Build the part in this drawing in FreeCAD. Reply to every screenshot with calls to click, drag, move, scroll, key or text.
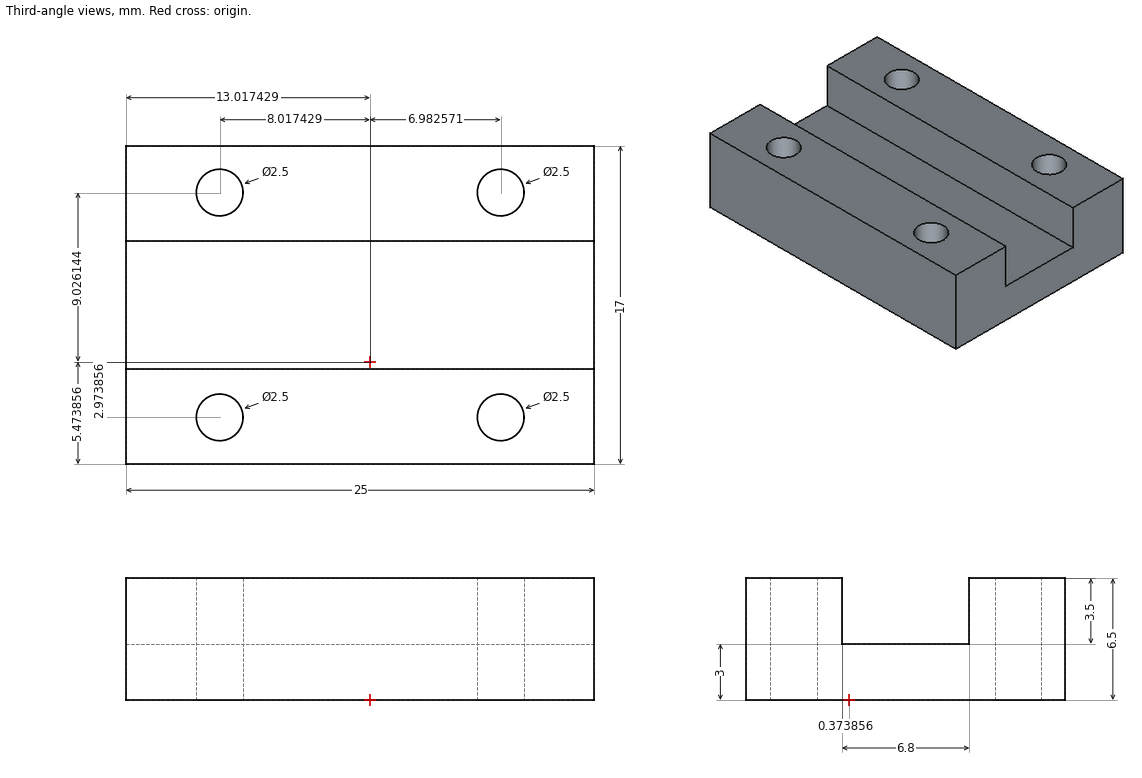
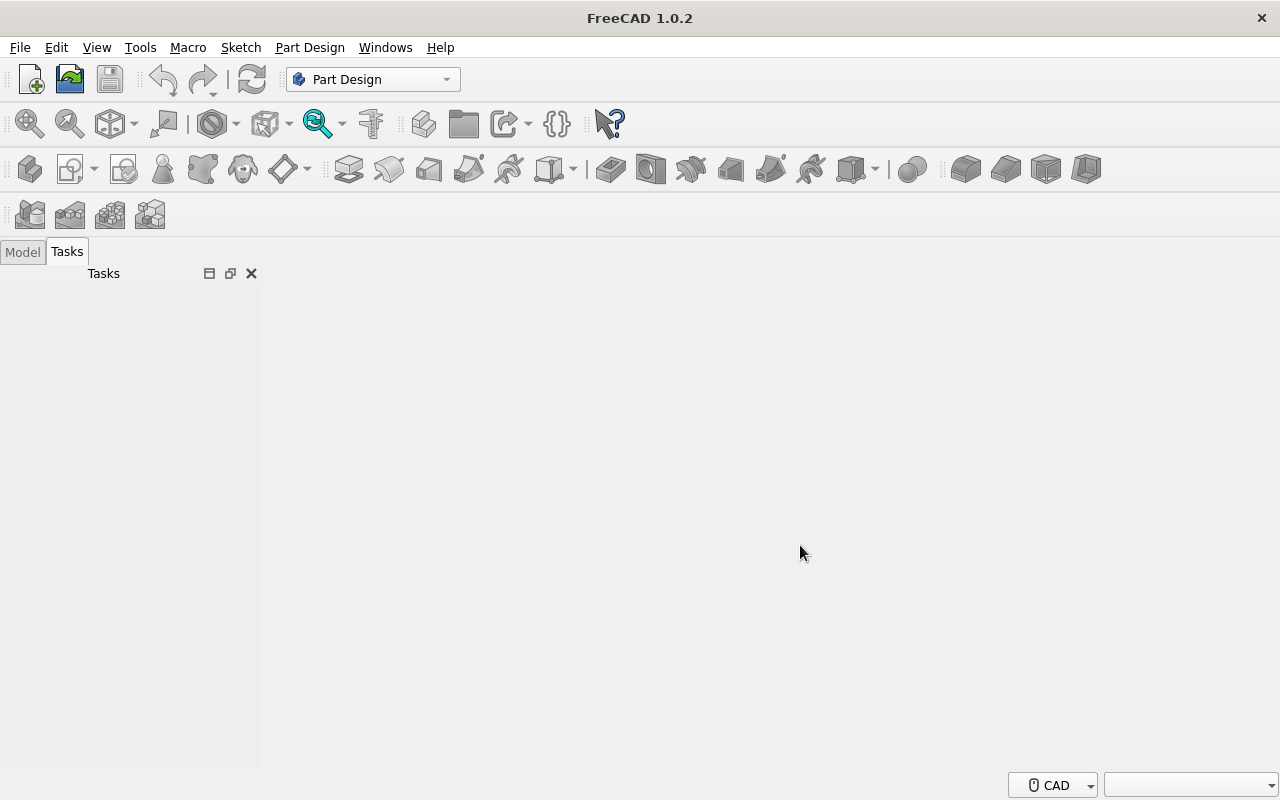
click(30, 80)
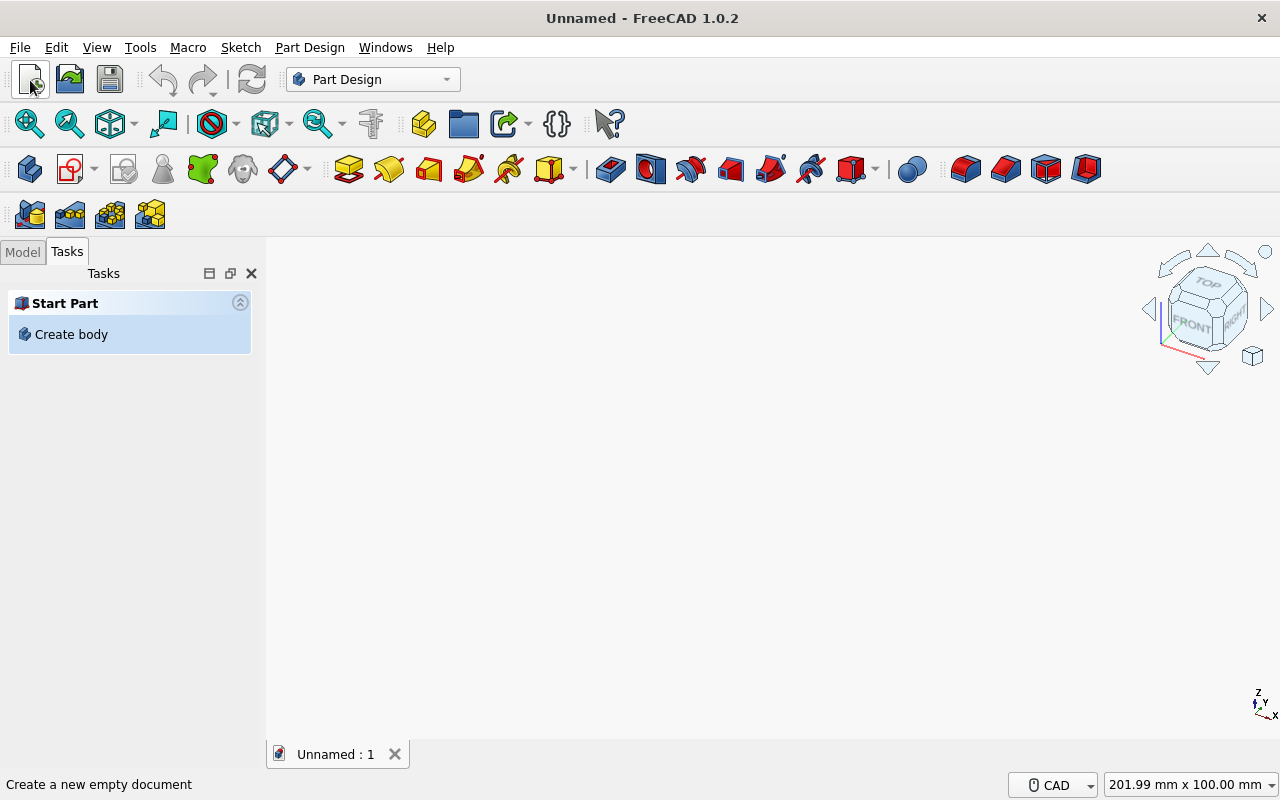
click(70, 170)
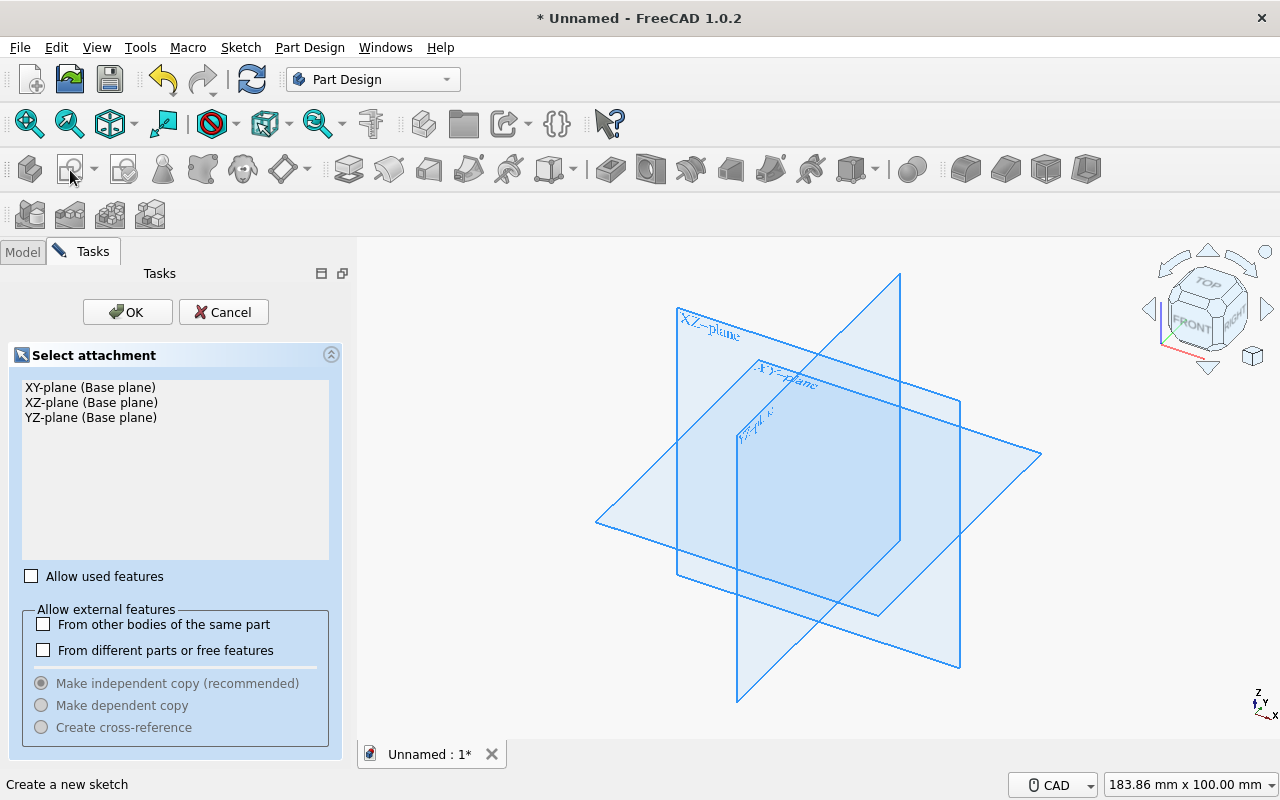
click(82, 388)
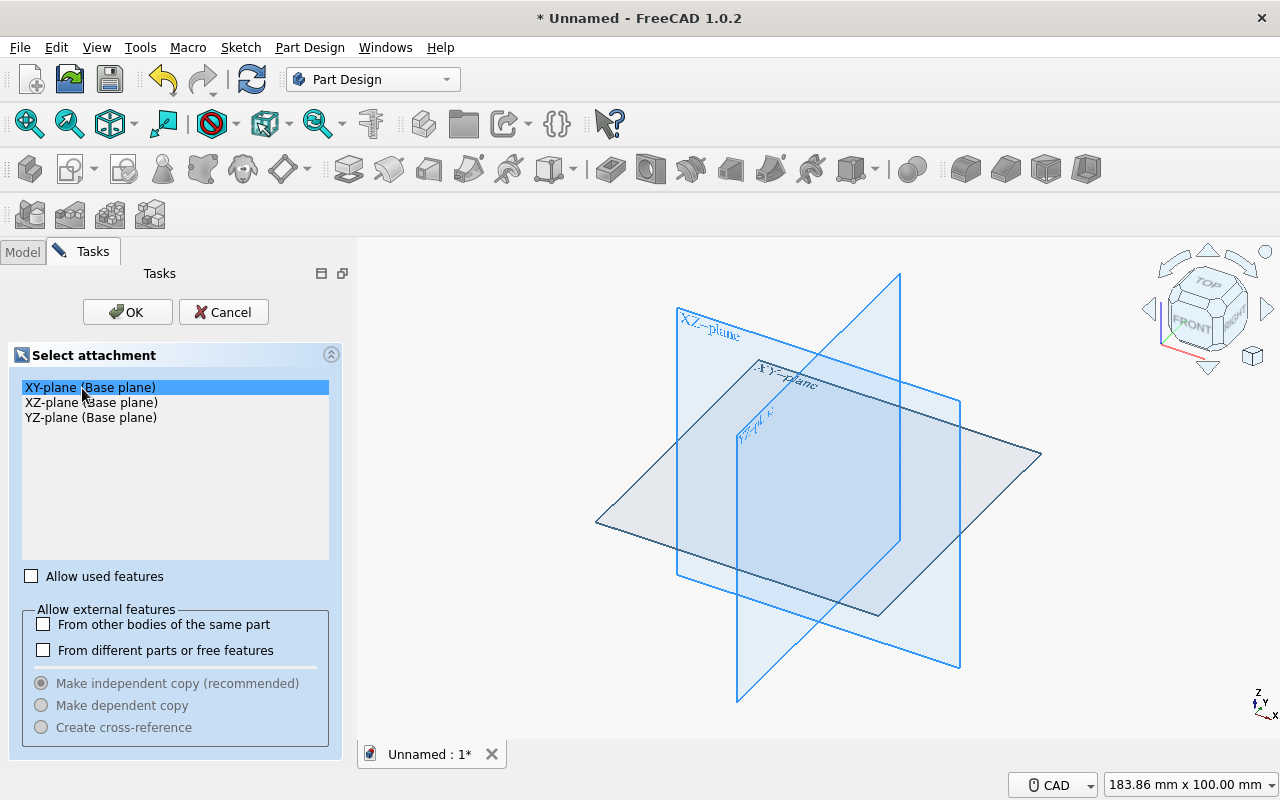
click(128, 312)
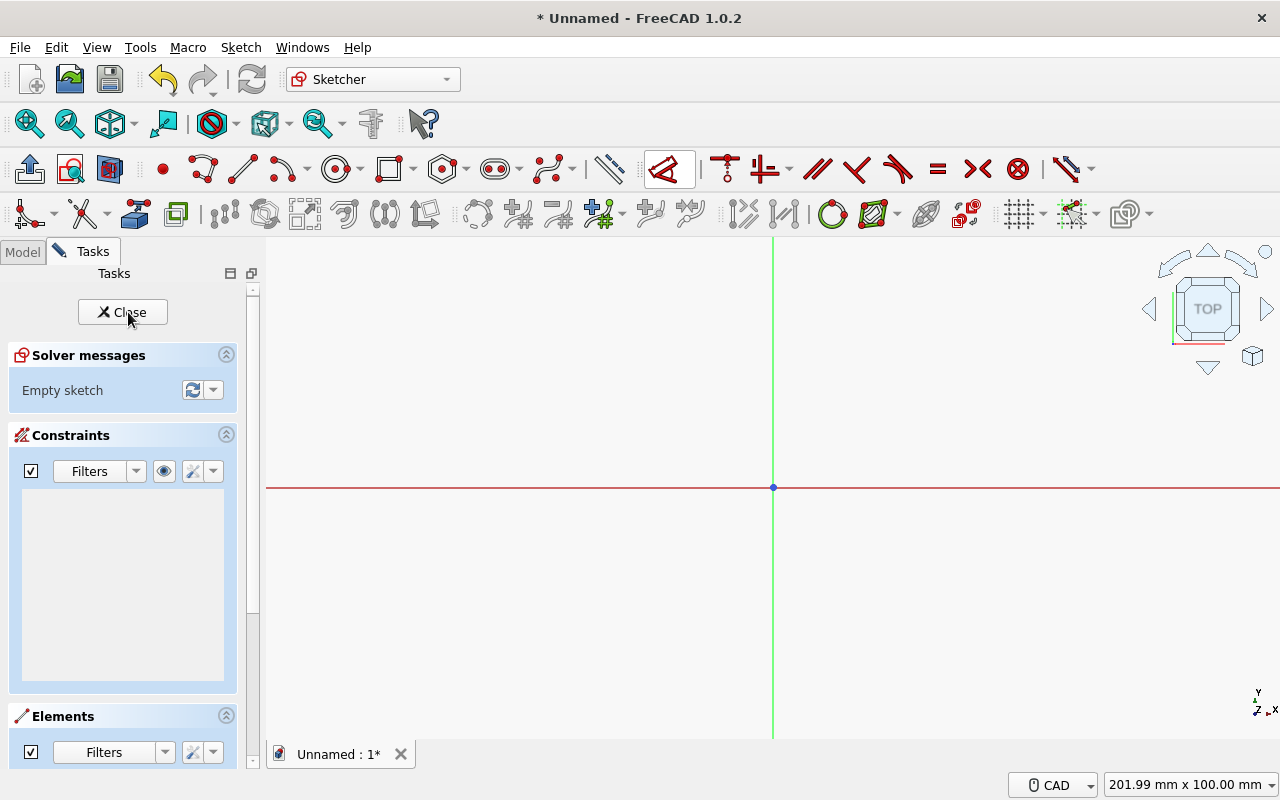
scroll(792, 468, up, 7)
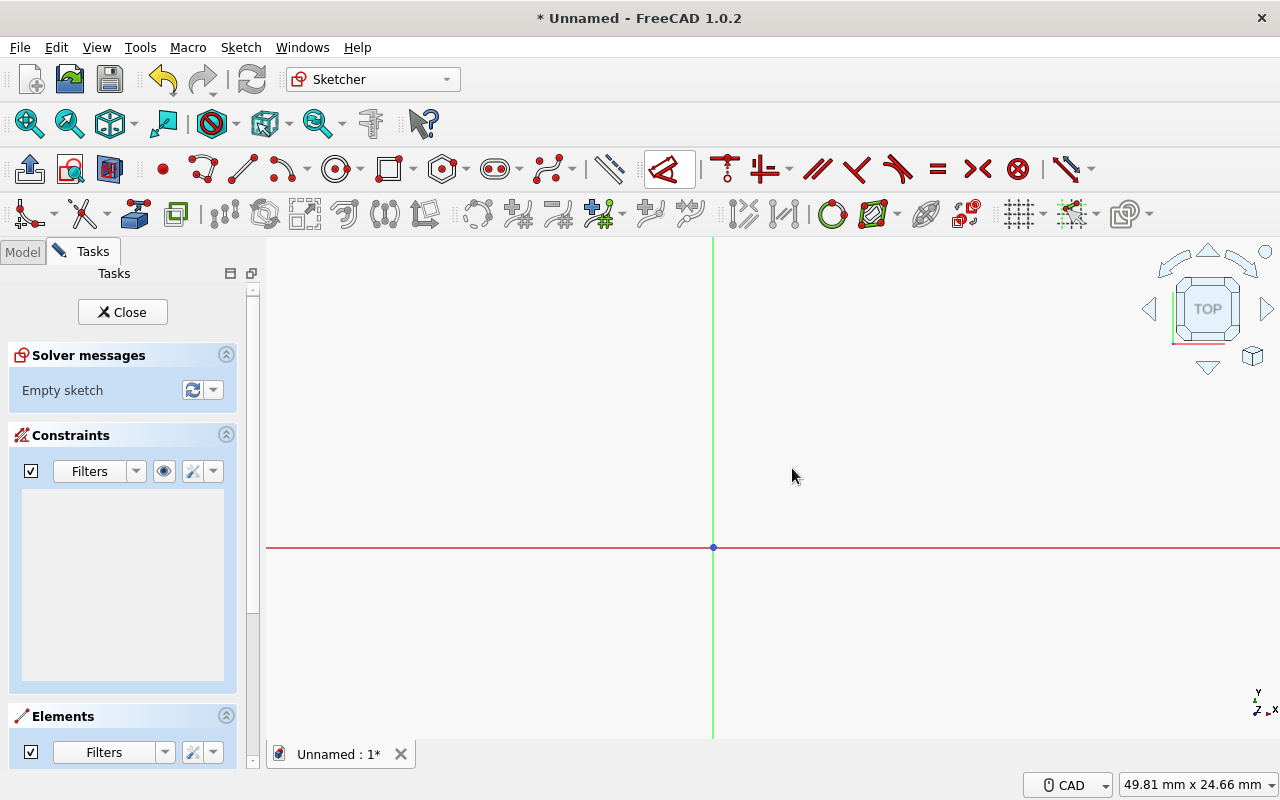
click(390, 170)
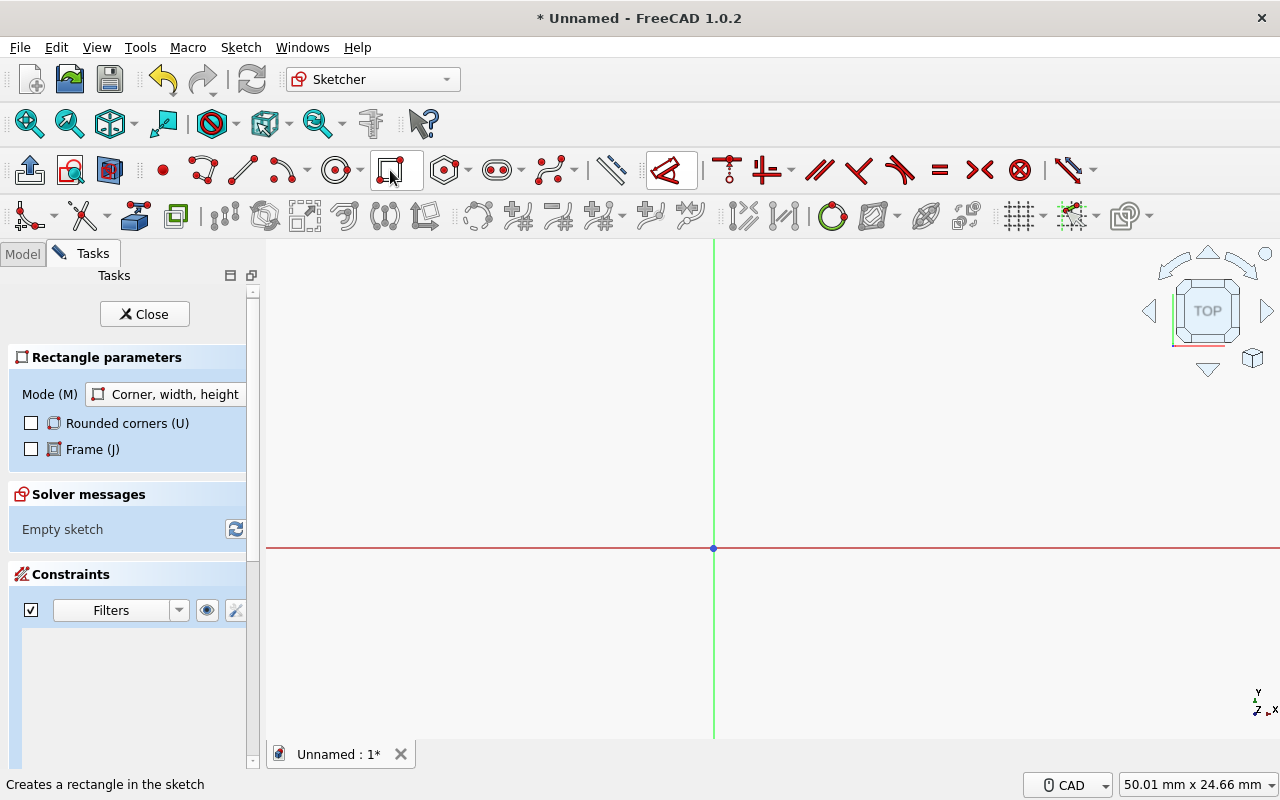
click(450, 315)
move(957, 659)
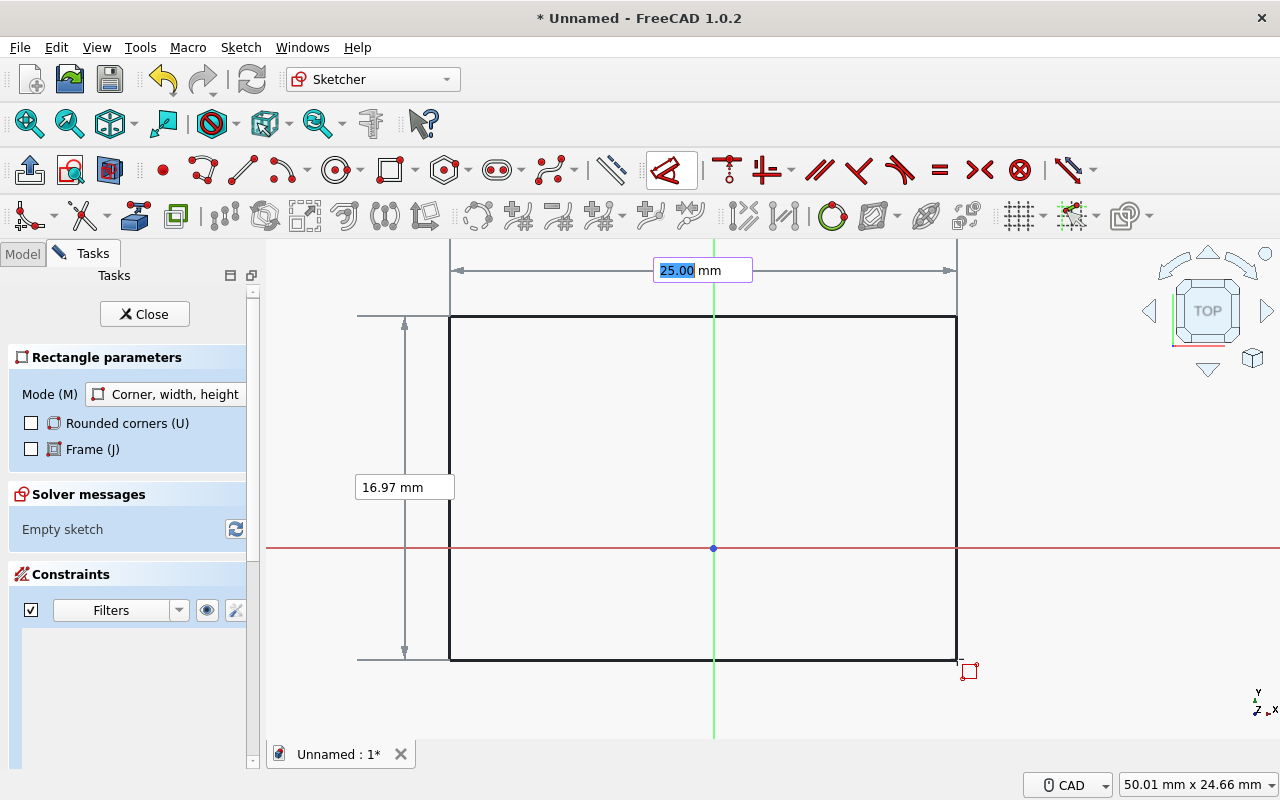
text(25)
key(Tab)
text(17)
key(Return)
key(Escape)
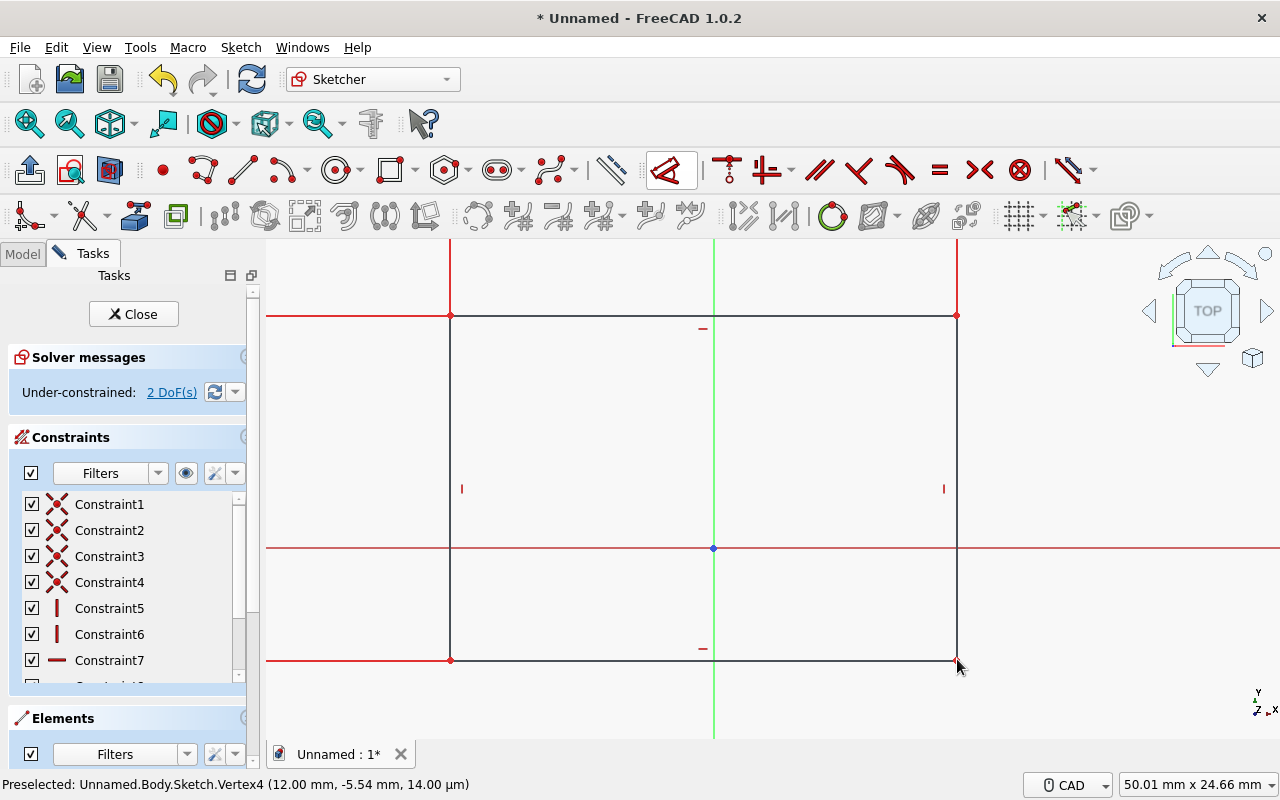
key(d)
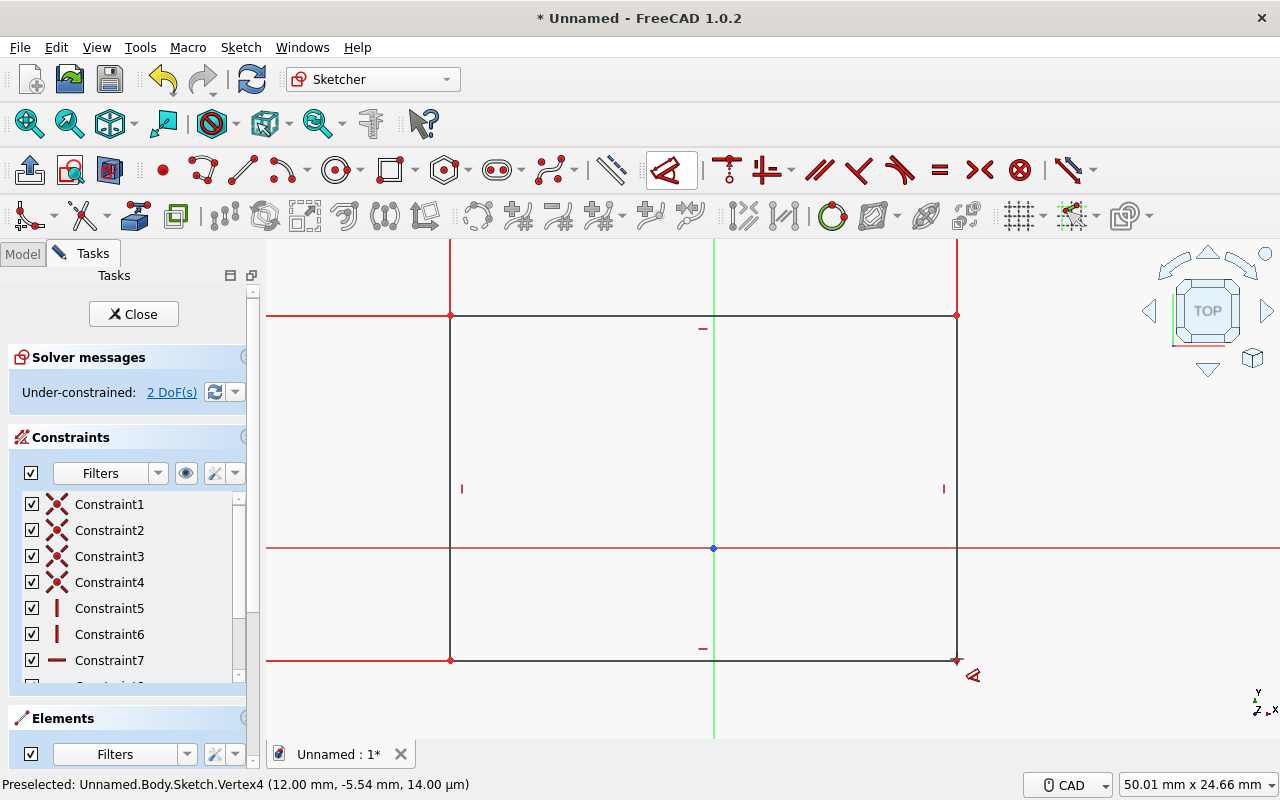
click(450, 661)
click(416, 605)